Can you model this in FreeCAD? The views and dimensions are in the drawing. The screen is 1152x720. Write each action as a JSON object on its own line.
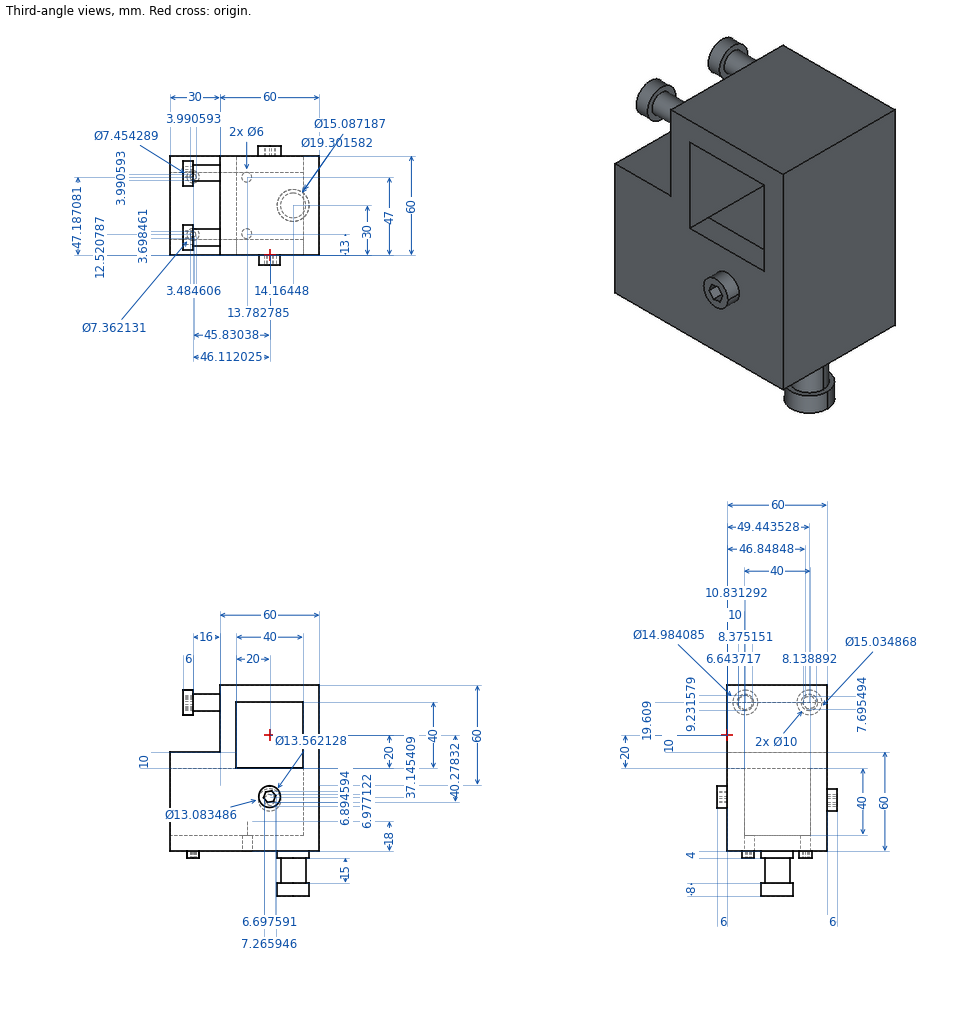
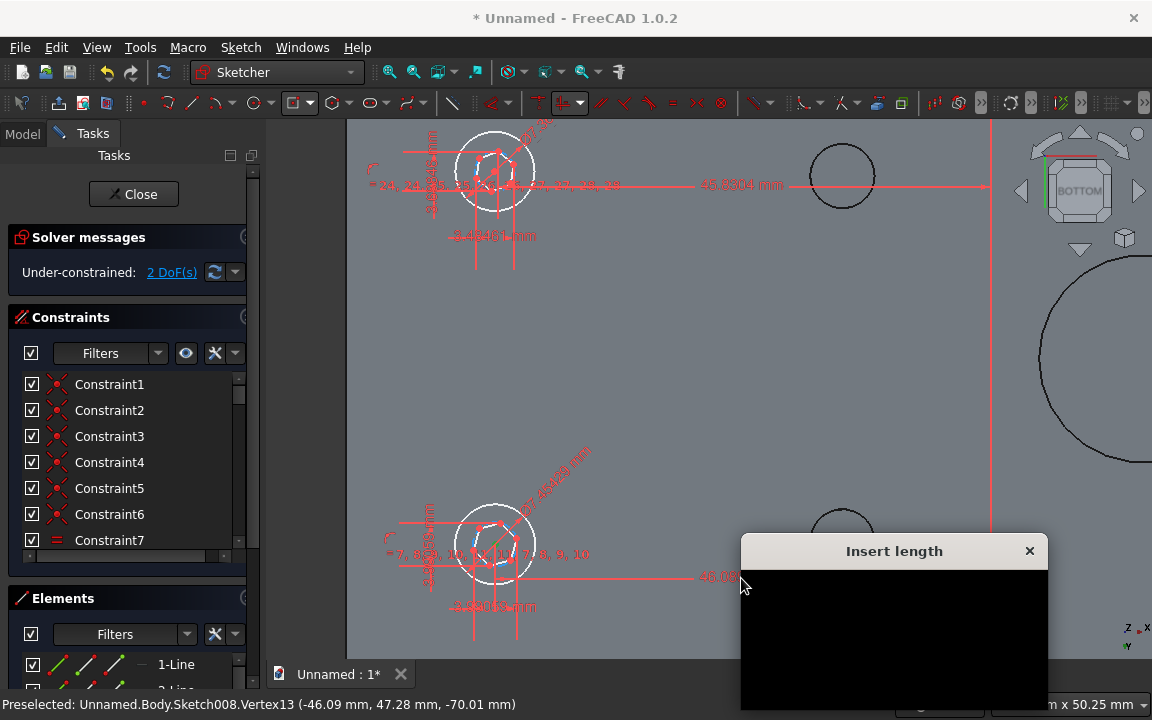
{"action": "type", "text": "46.112025"}
{"action": "key", "text": "Return"}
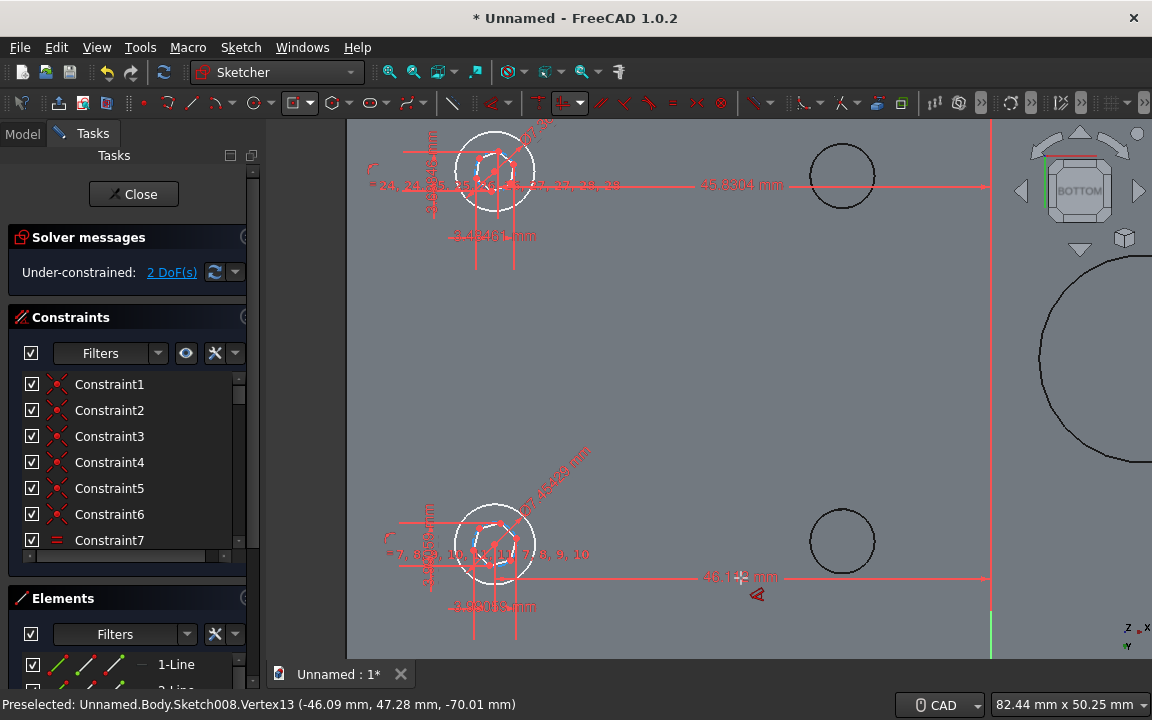
{"action": "left_click", "coordinate": [495, 544]}
{"action": "left_click", "coordinate": [461, 346]}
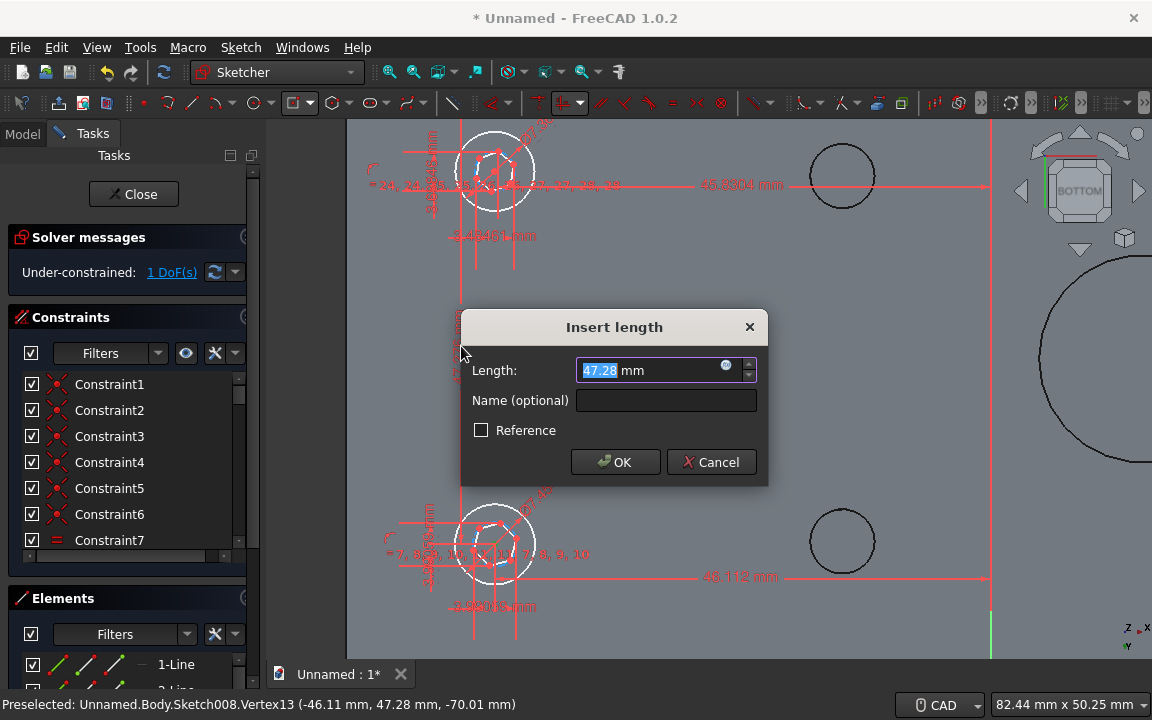
{"action": "type", "text": "47.187081"}
{"action": "key", "text": "Return"}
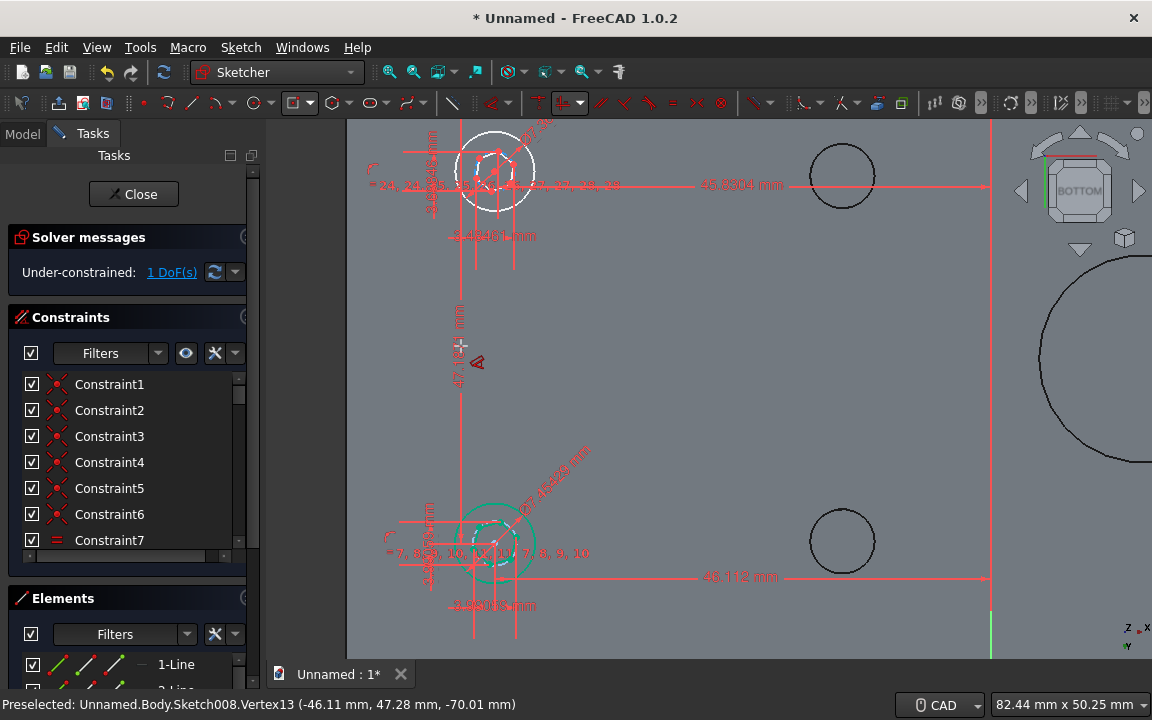
{"action": "left_click", "coordinate": [495, 171]}
{"action": "left_click", "coordinate": [437, 151]}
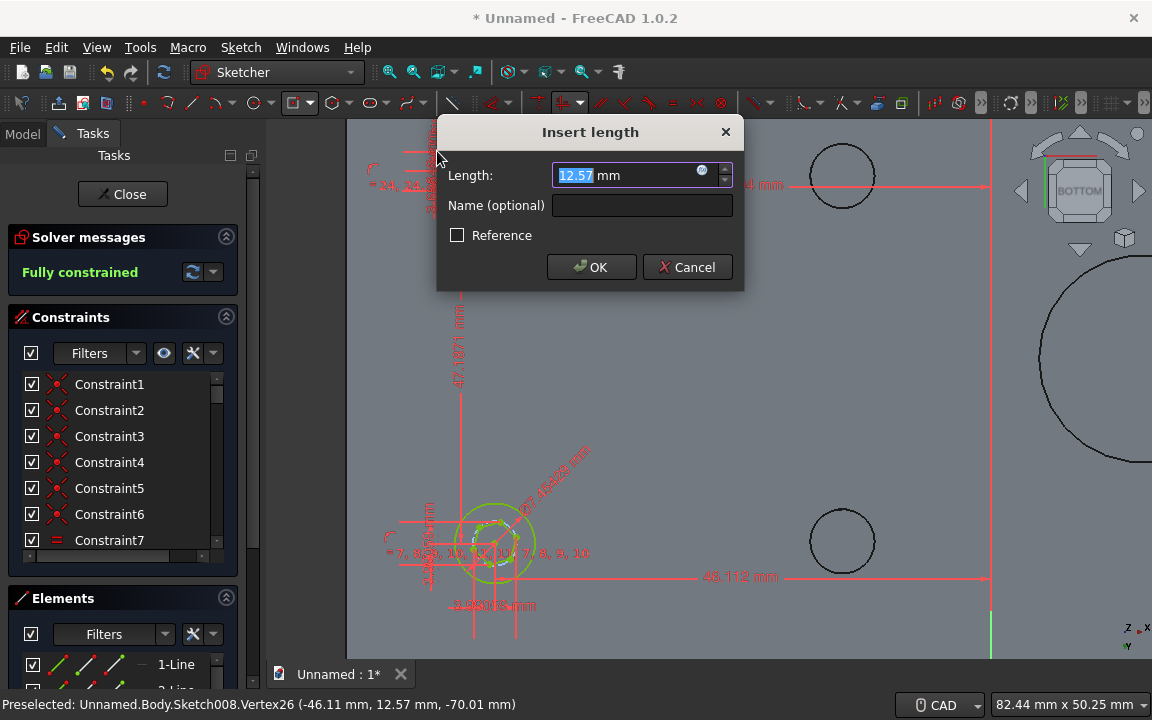
{"action": "type", "text": "12.520787"}
{"action": "key", "text": "Return"}
{"action": "key", "text": "Escape"}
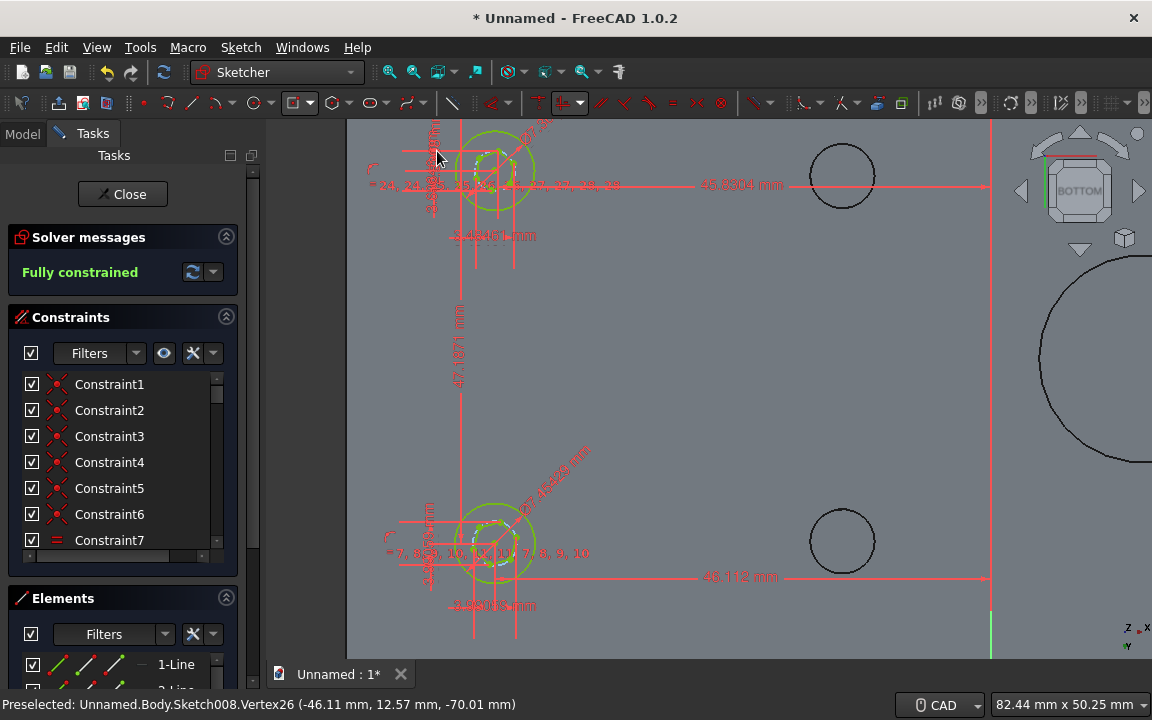
{"action": "left_click", "coordinate": [123, 194]}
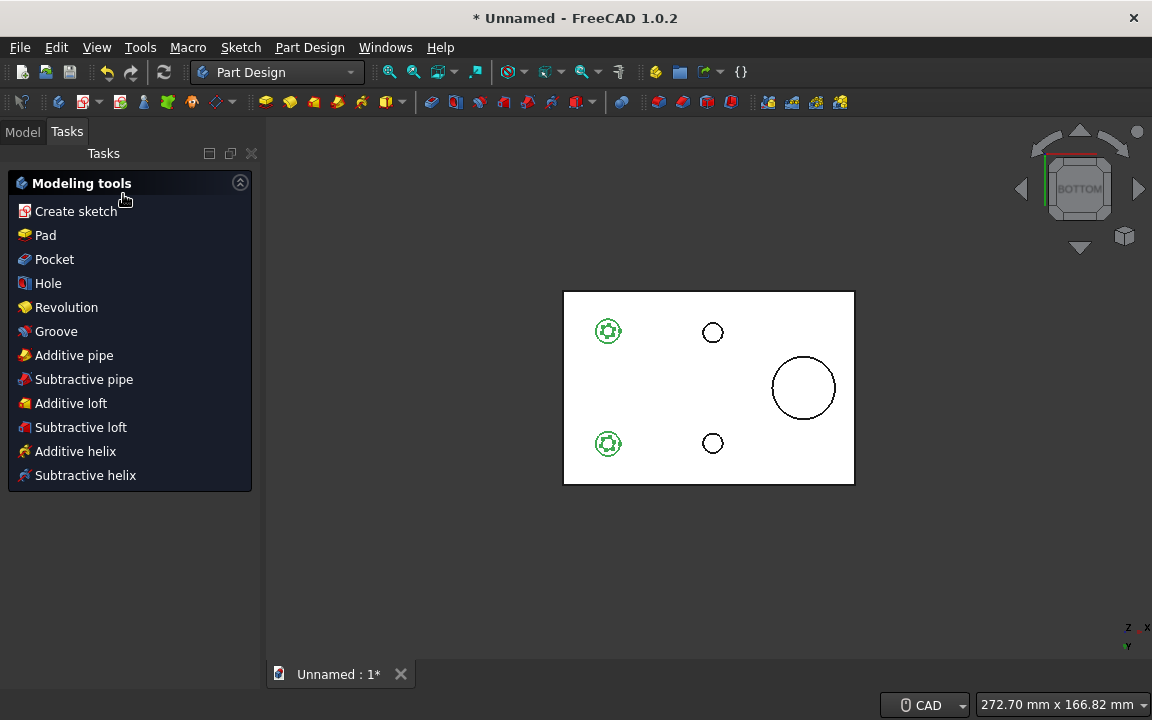
{"action": "left_click", "coordinate": [266, 102]}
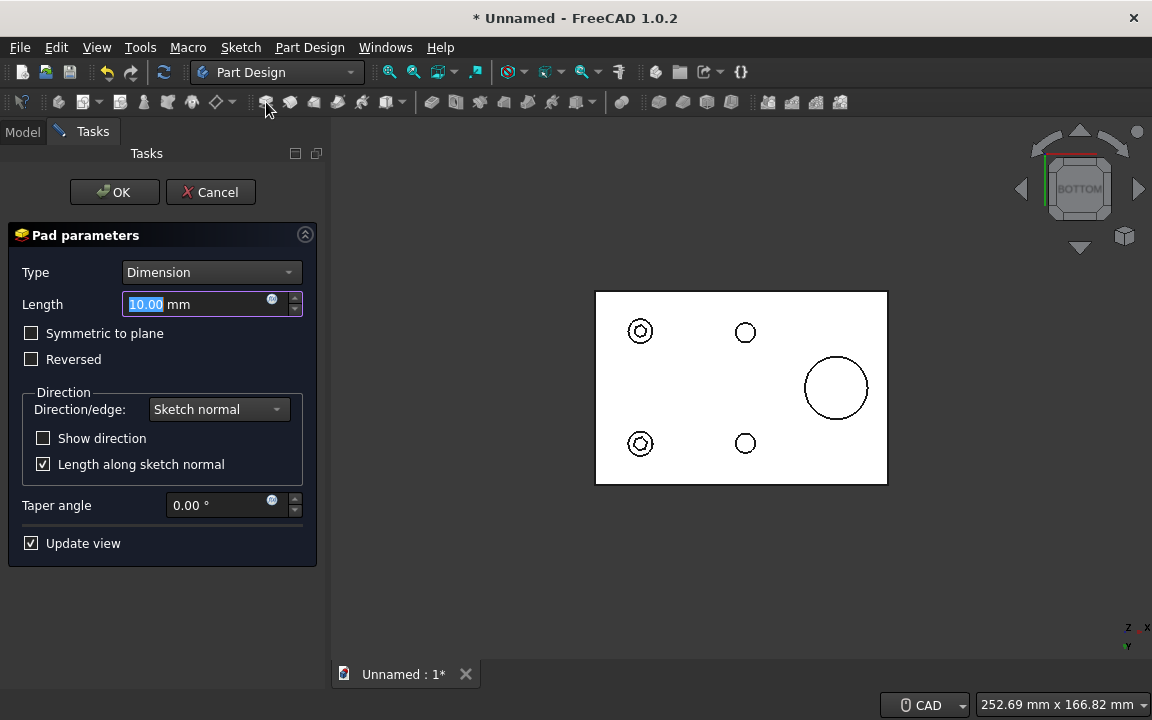
{"action": "type", "text": "4"}
{"action": "key", "text": "Tab"}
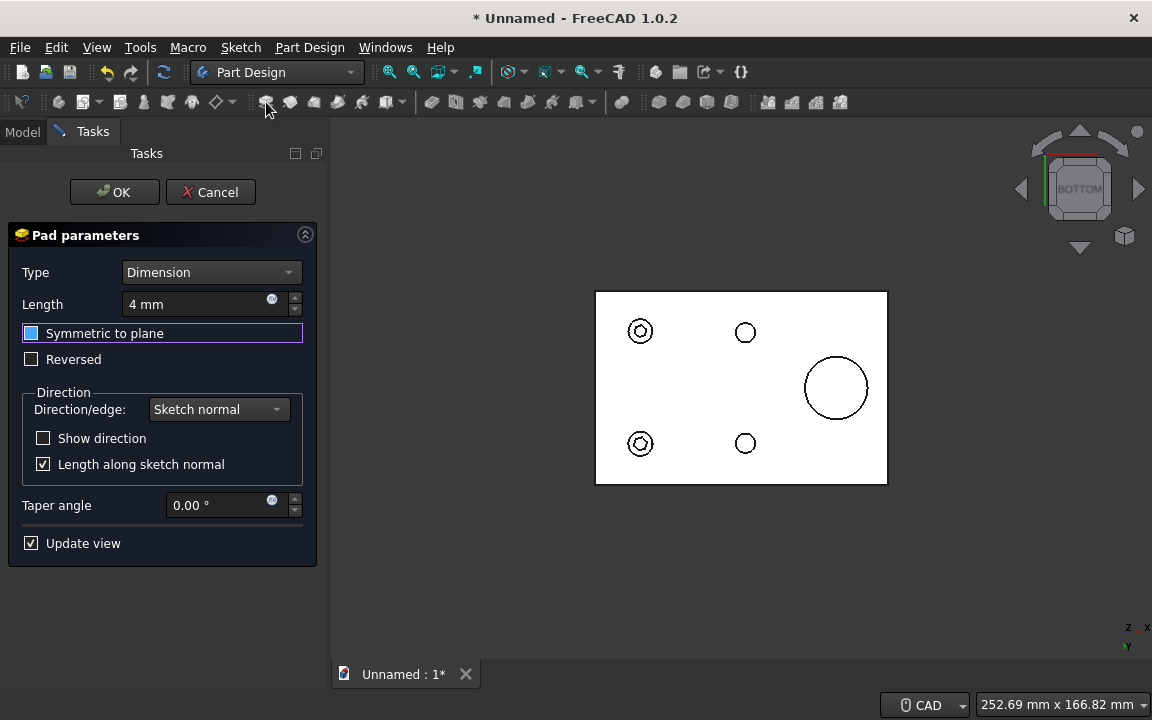
{"action": "left_click", "coordinate": [115, 192]}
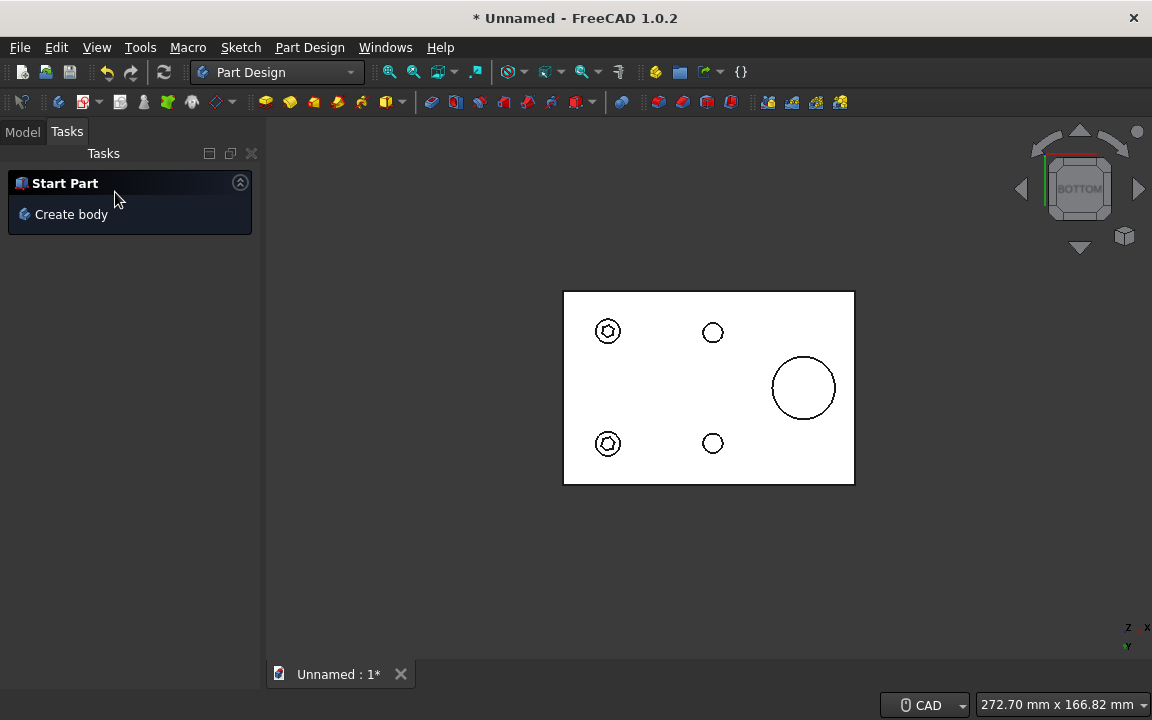
{"action": "left_click", "coordinate": [390, 72]}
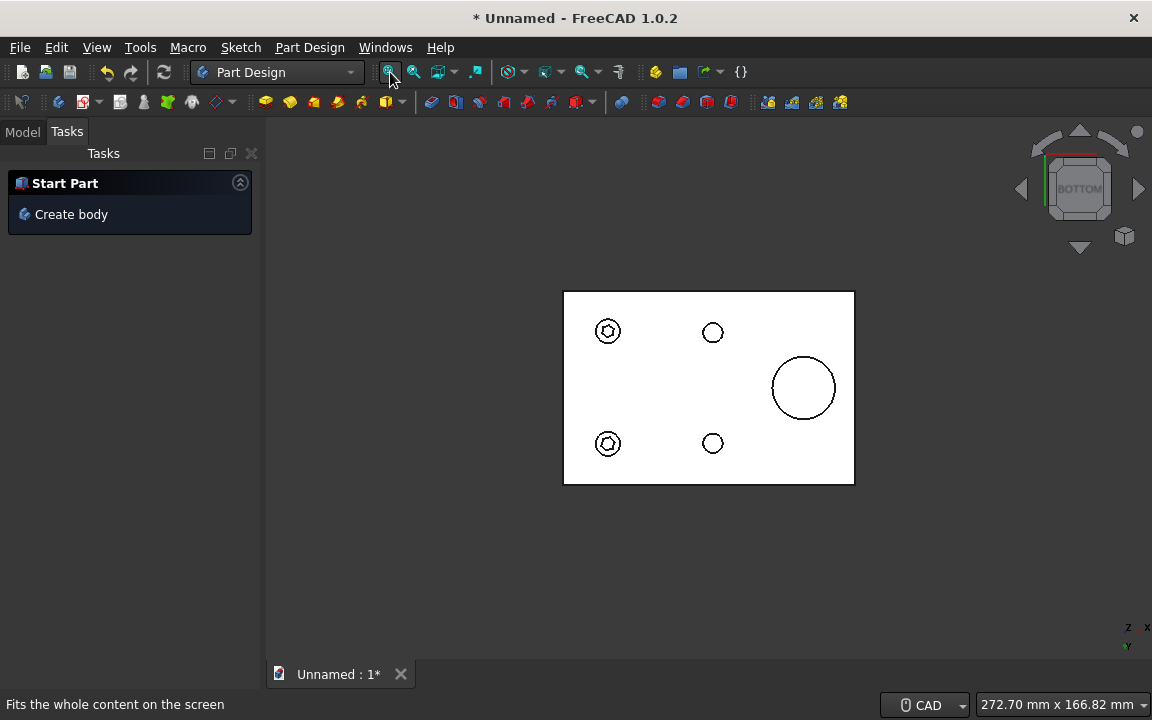
{"action": "key", "text": "4"}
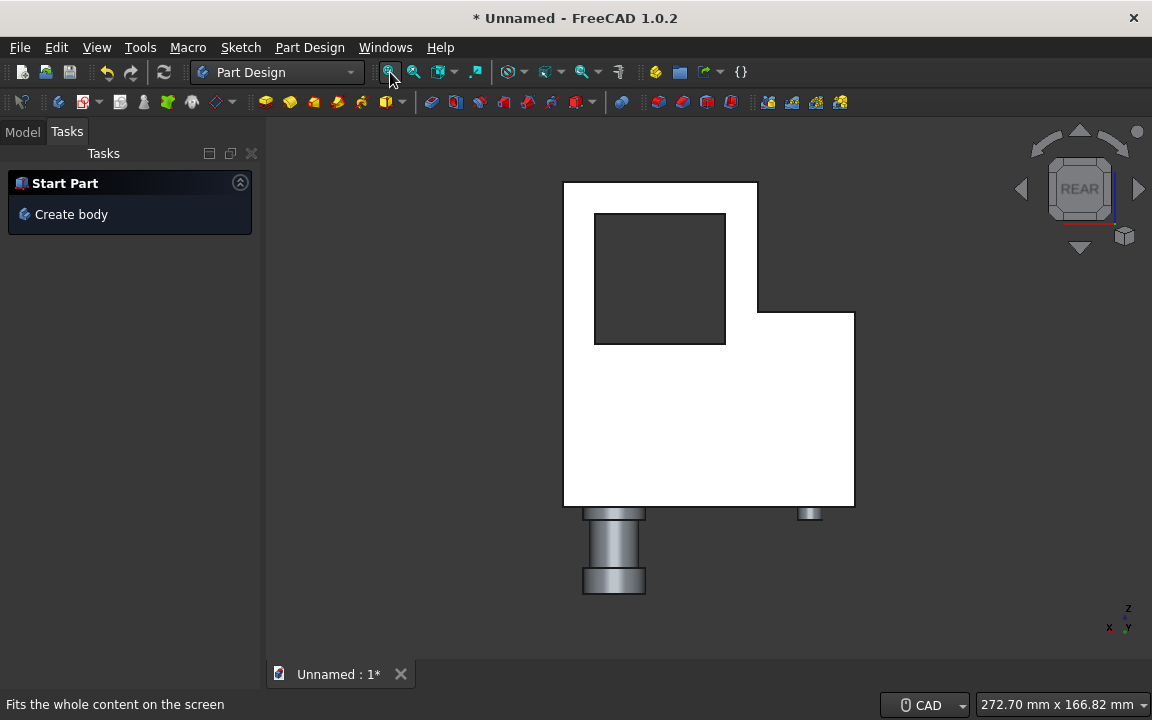
{"action": "left_click", "coordinate": [667, 436]}